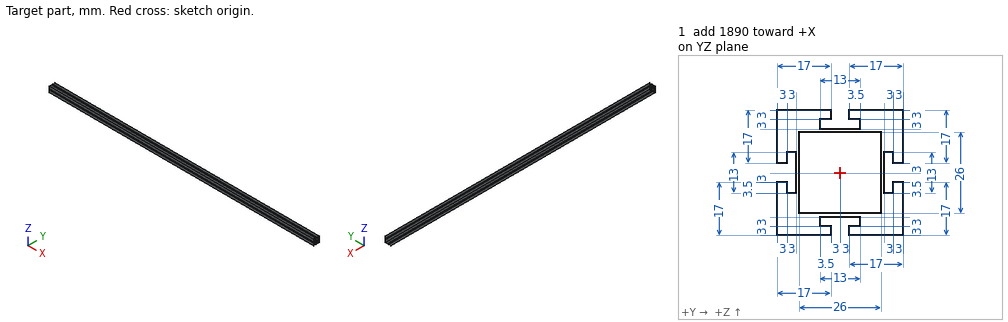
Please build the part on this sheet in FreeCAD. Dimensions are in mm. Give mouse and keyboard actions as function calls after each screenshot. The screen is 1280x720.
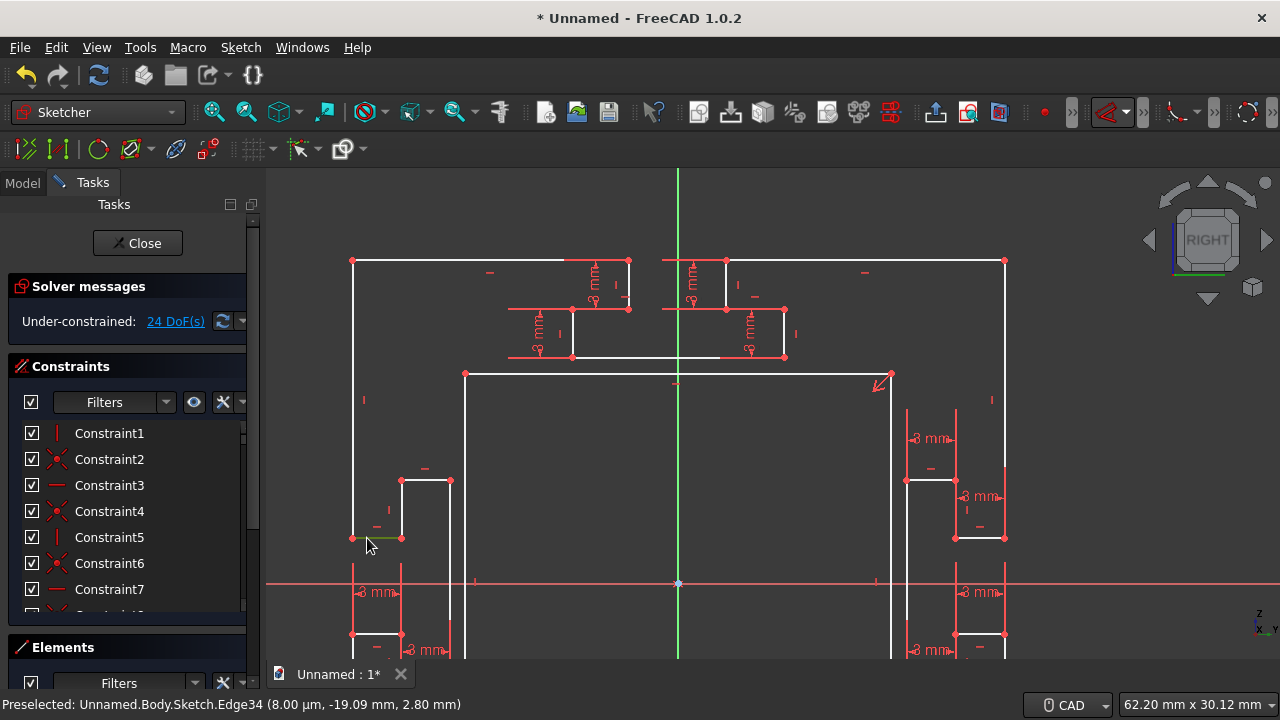
key(l)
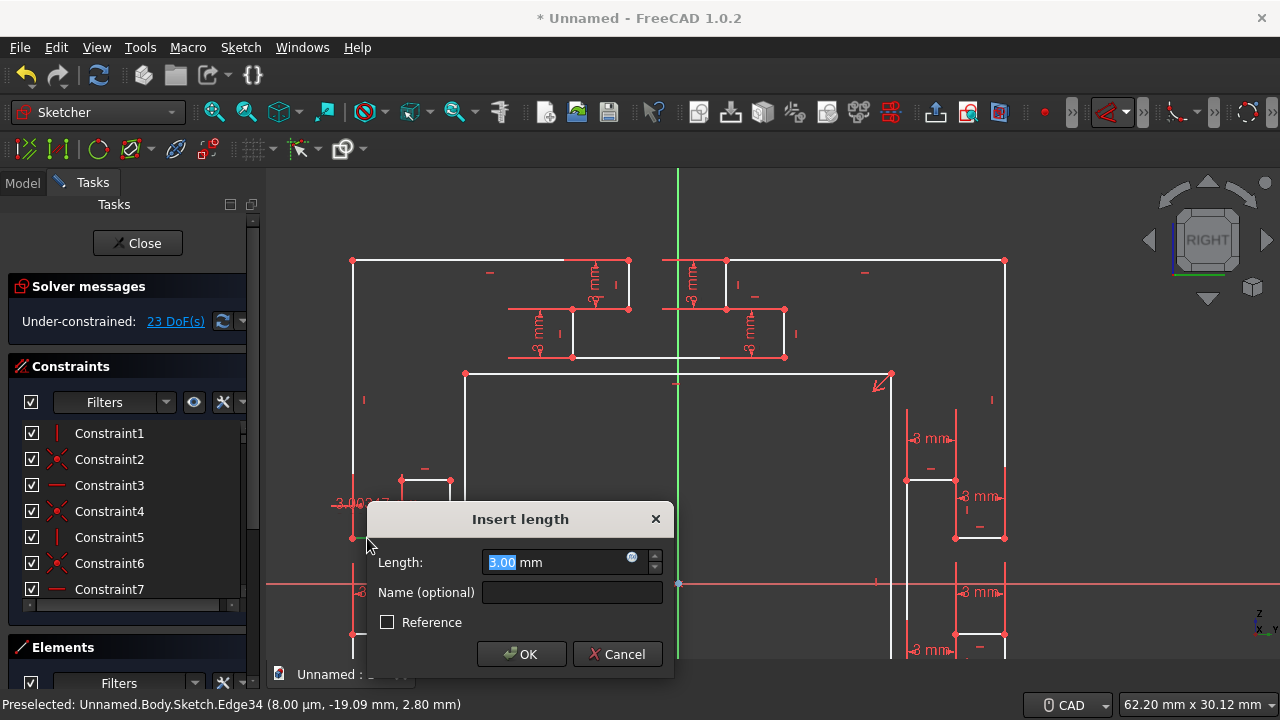
text(3)
key(Return)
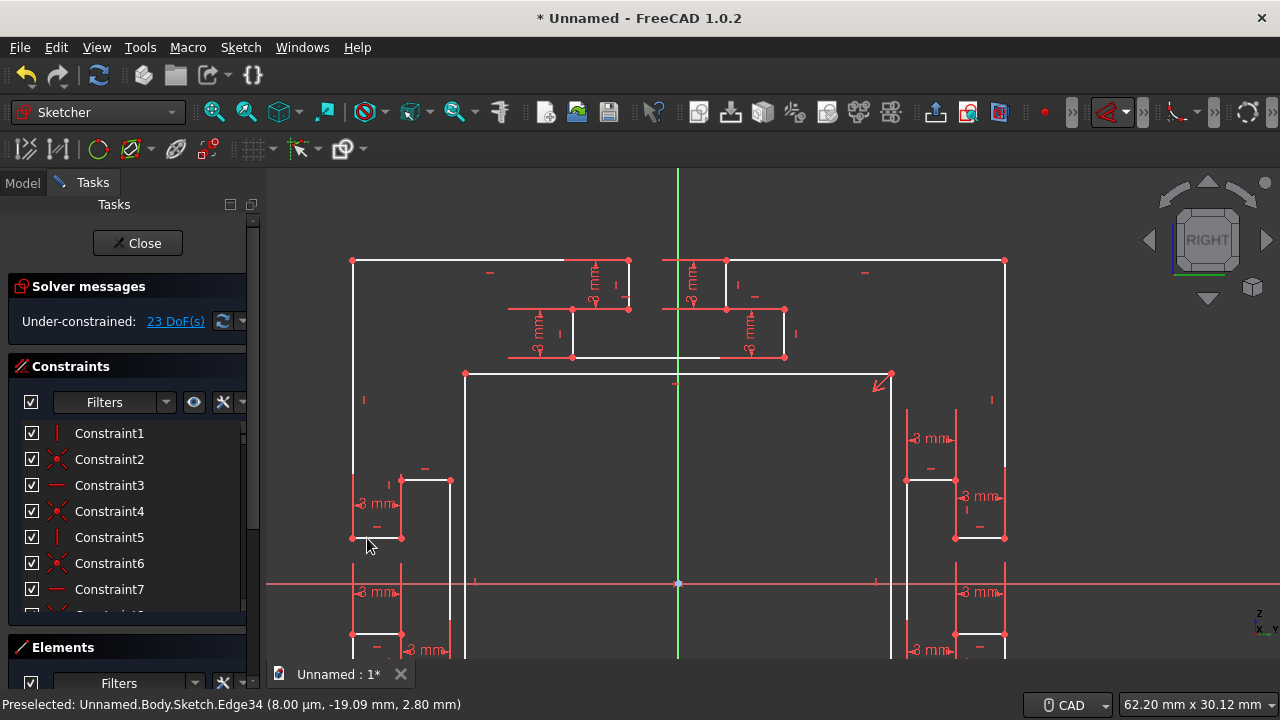
click(416, 480)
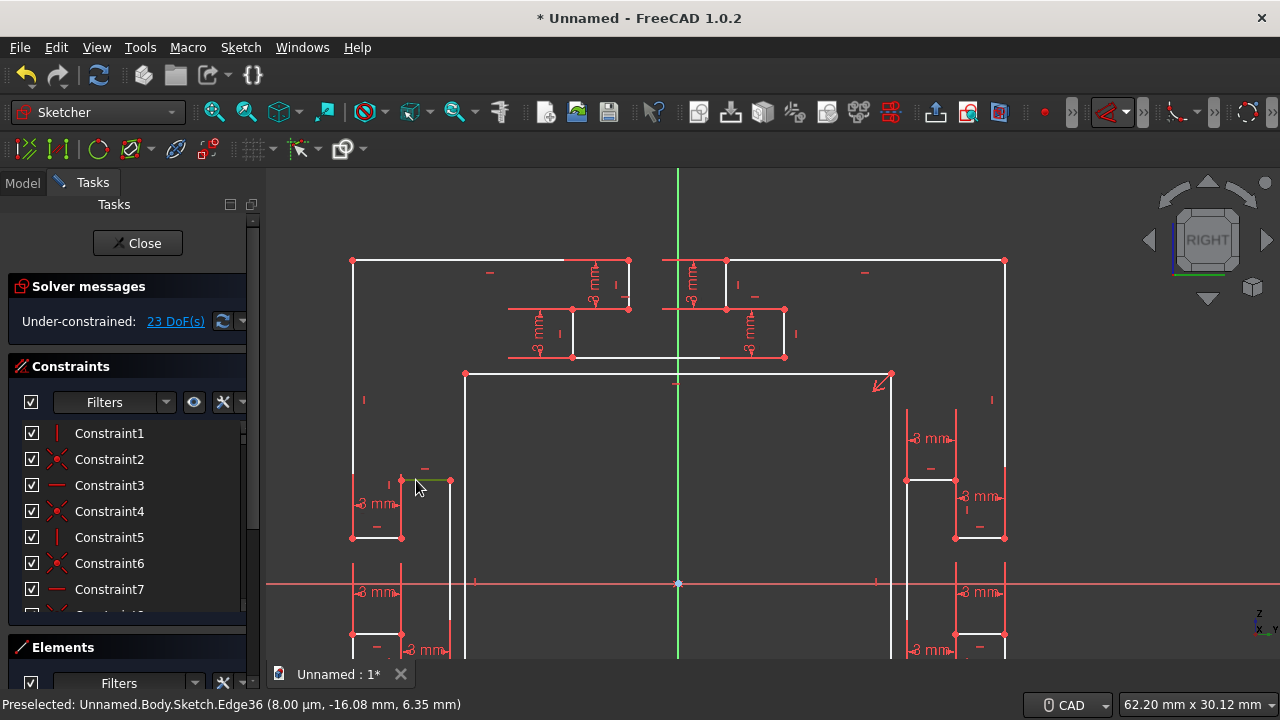
key(l)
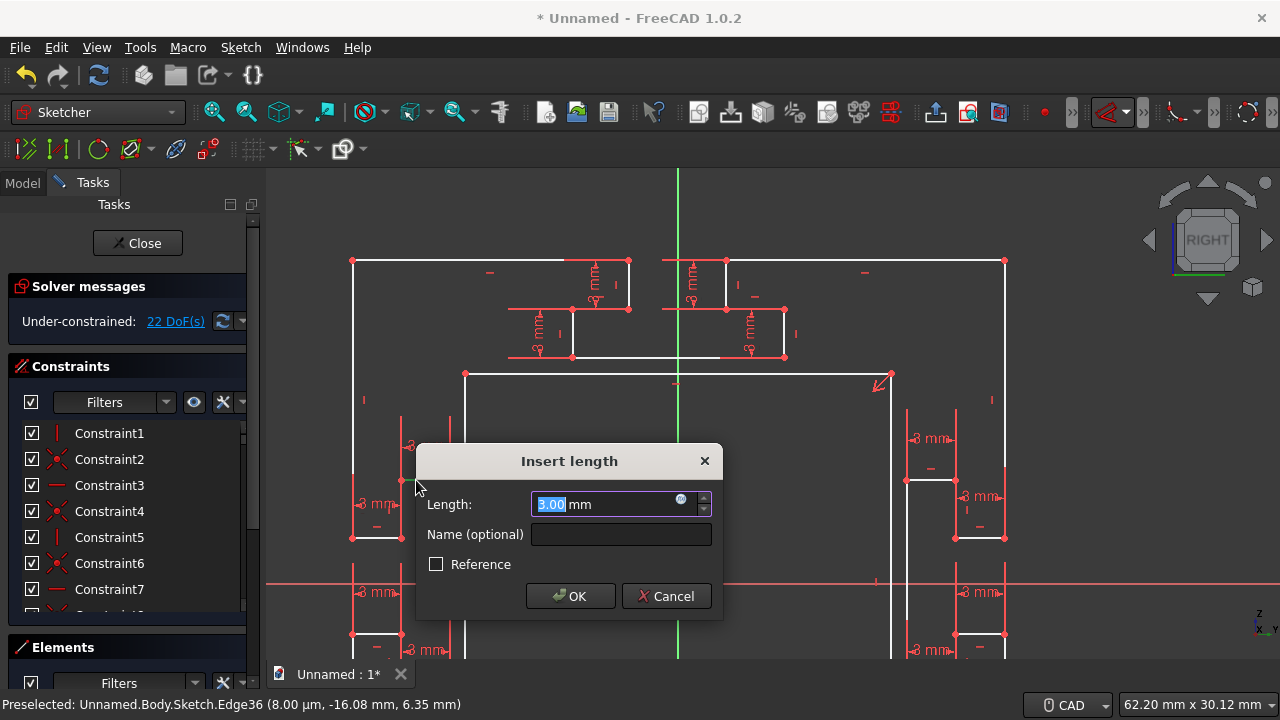
text(3)
key(Return)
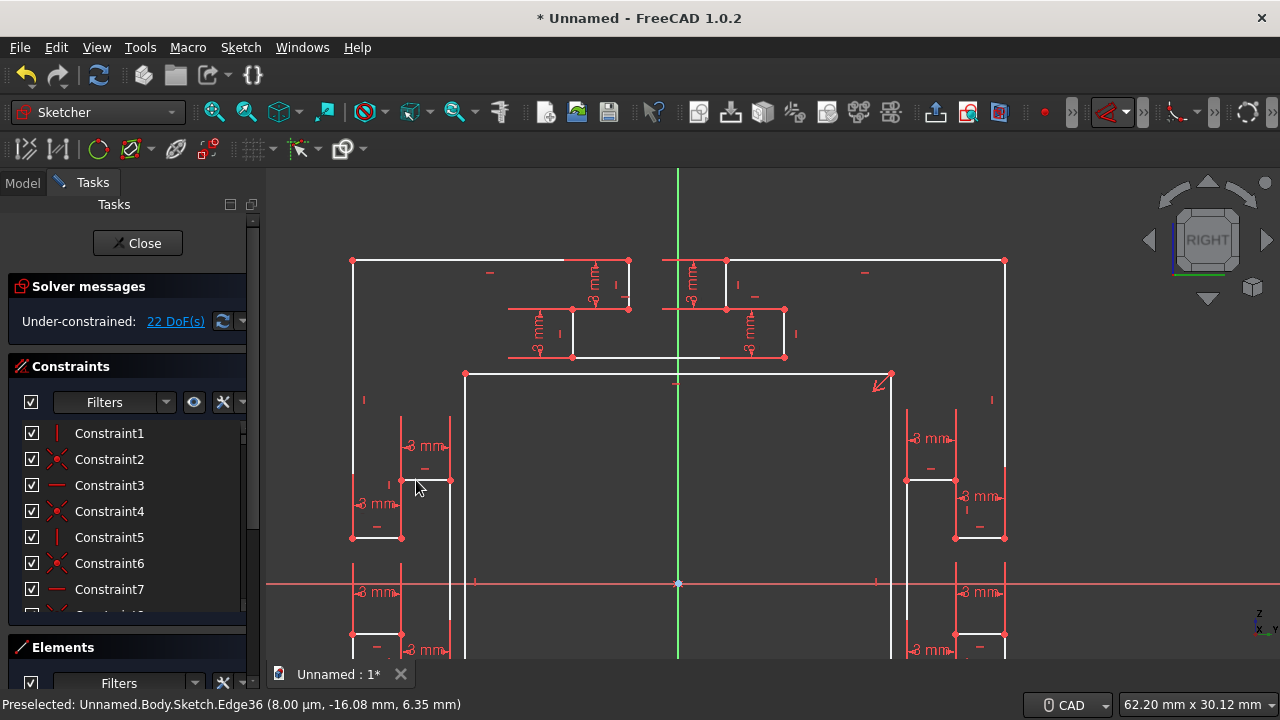
click(450, 544)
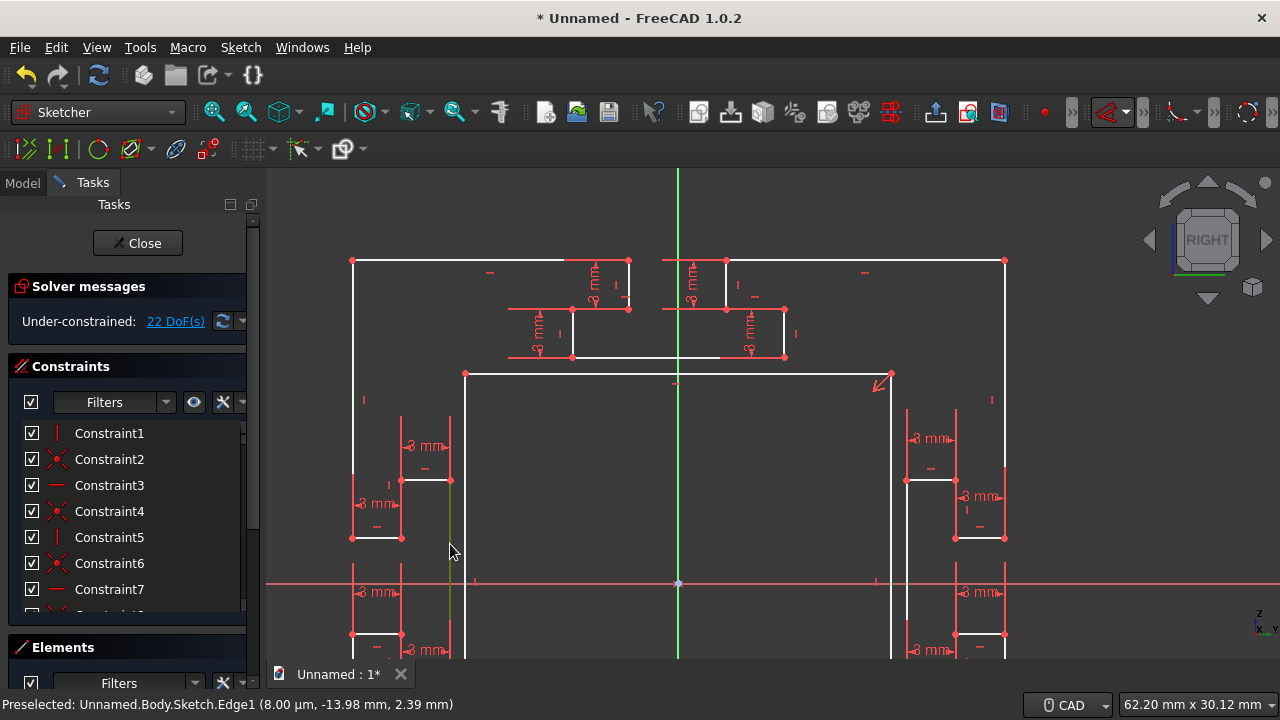
click(1128, 112)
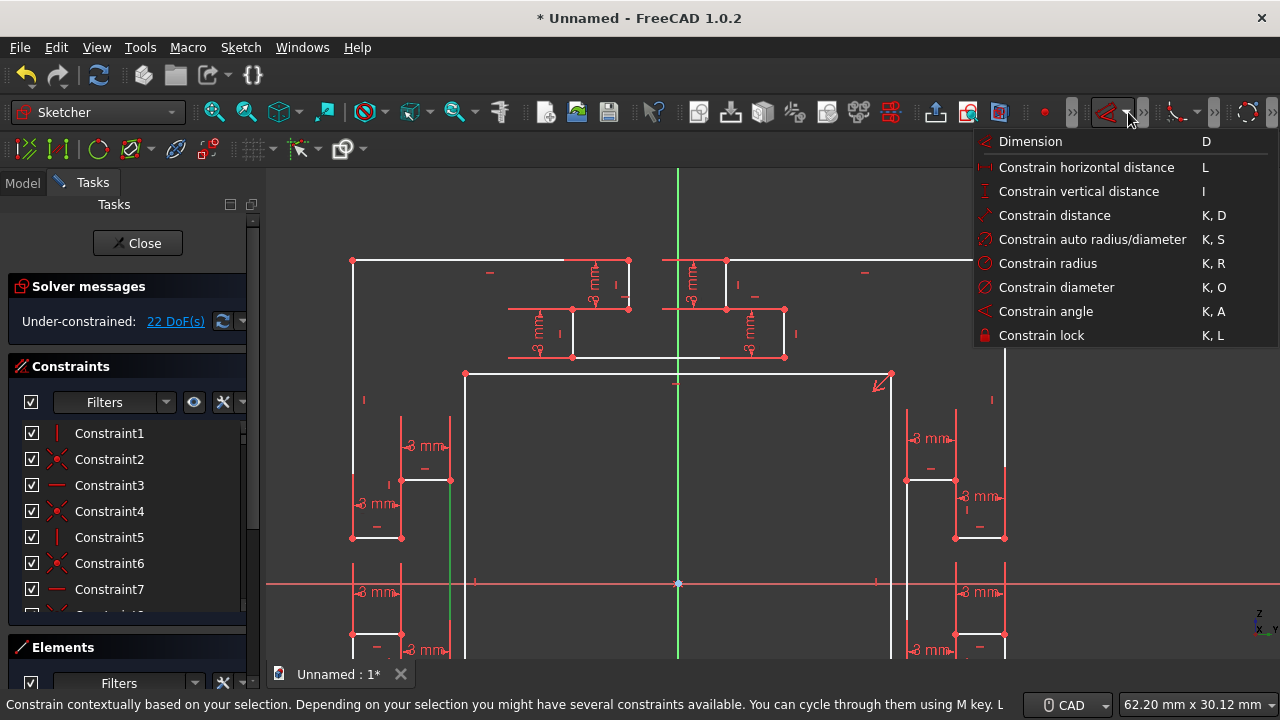
click(1126, 191)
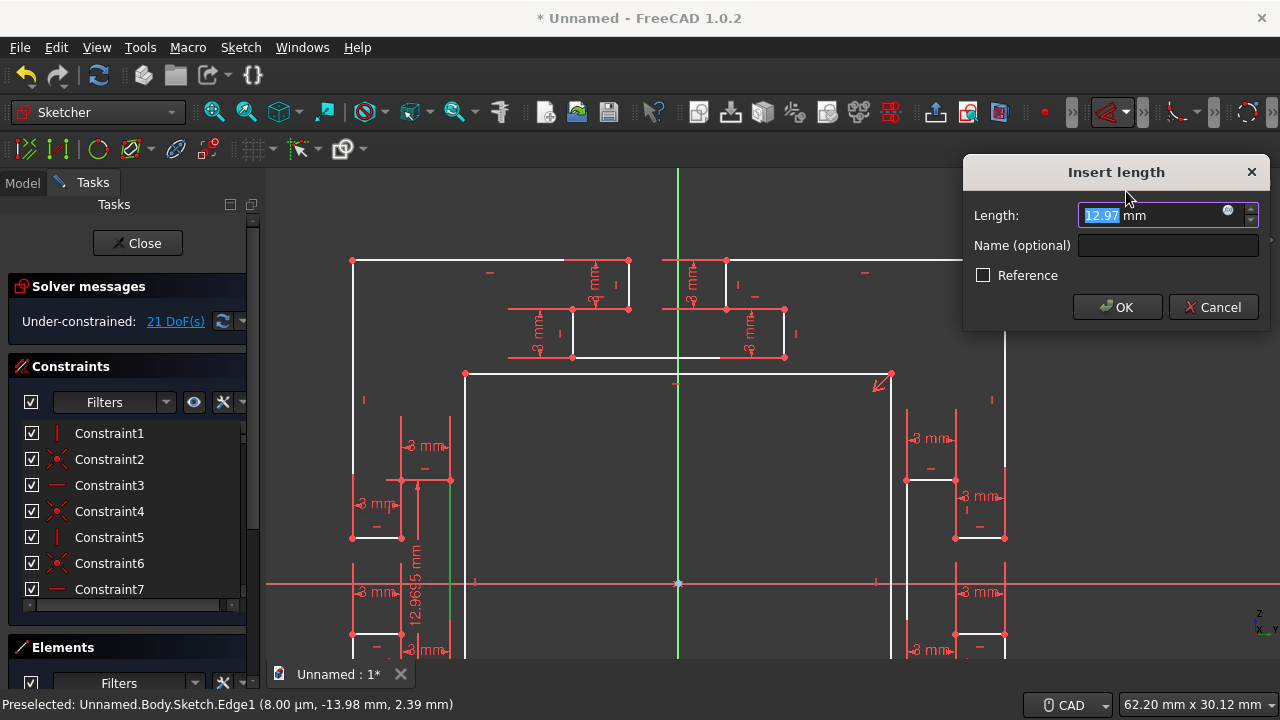
text(13)
key(Return)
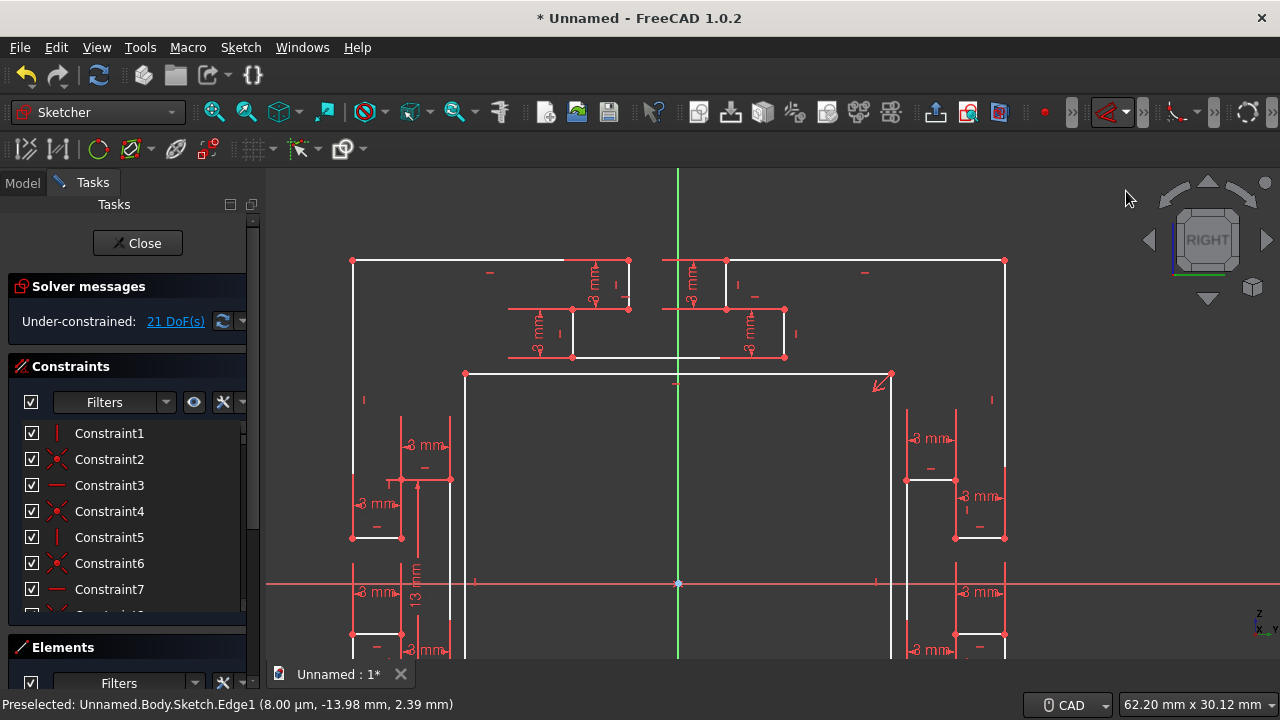
scroll(726, 274, down, 4)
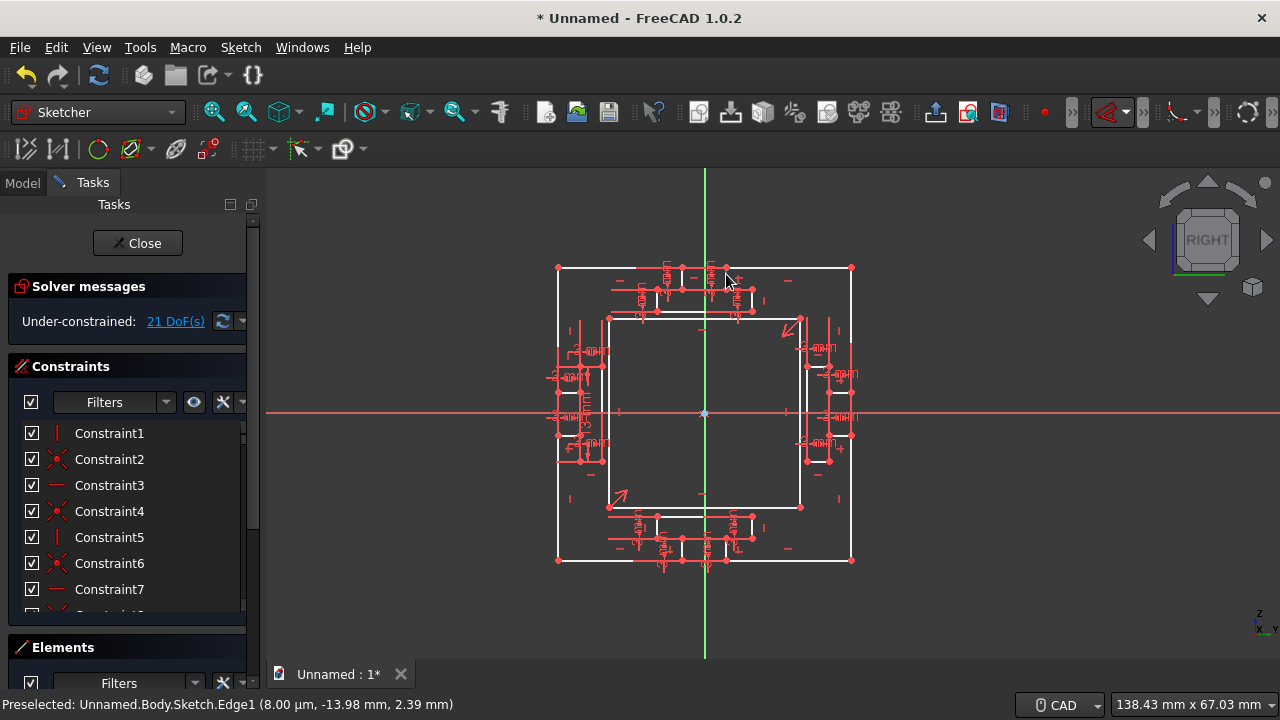
click(558, 473)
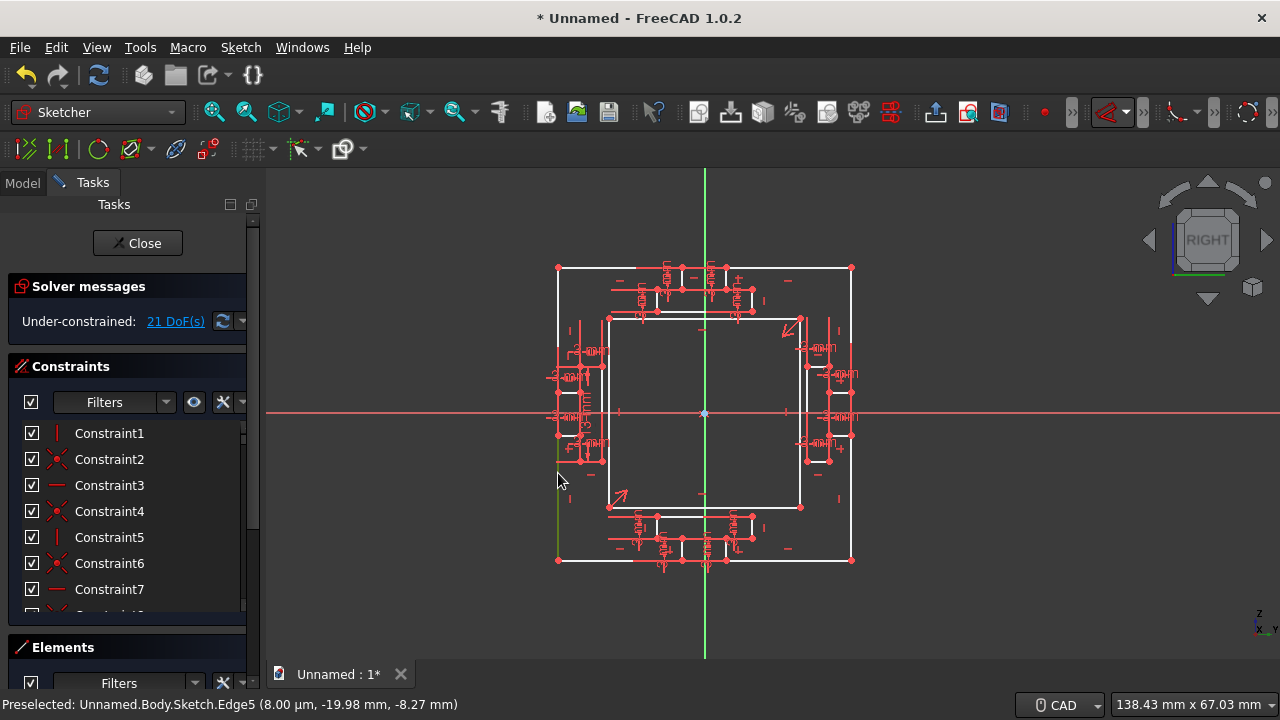
key(i)